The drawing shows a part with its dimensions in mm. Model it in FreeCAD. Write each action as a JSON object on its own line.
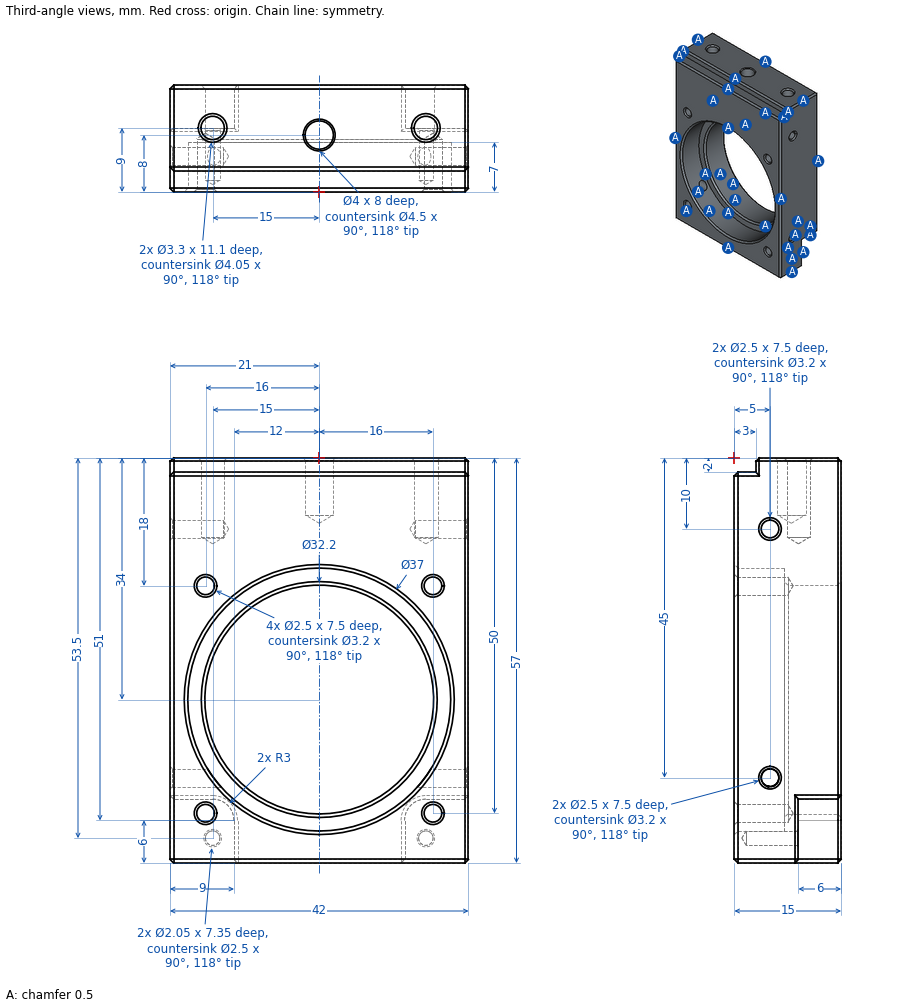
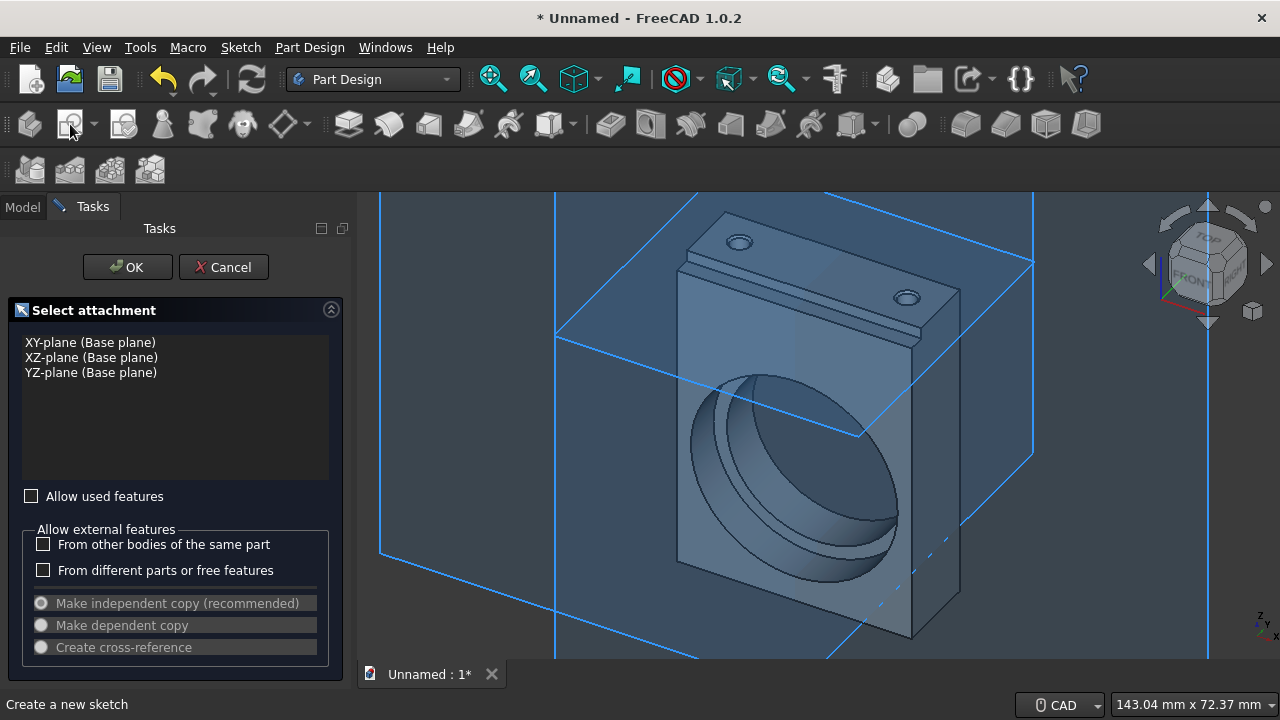
{"action": "left_click", "coordinate": [82, 342]}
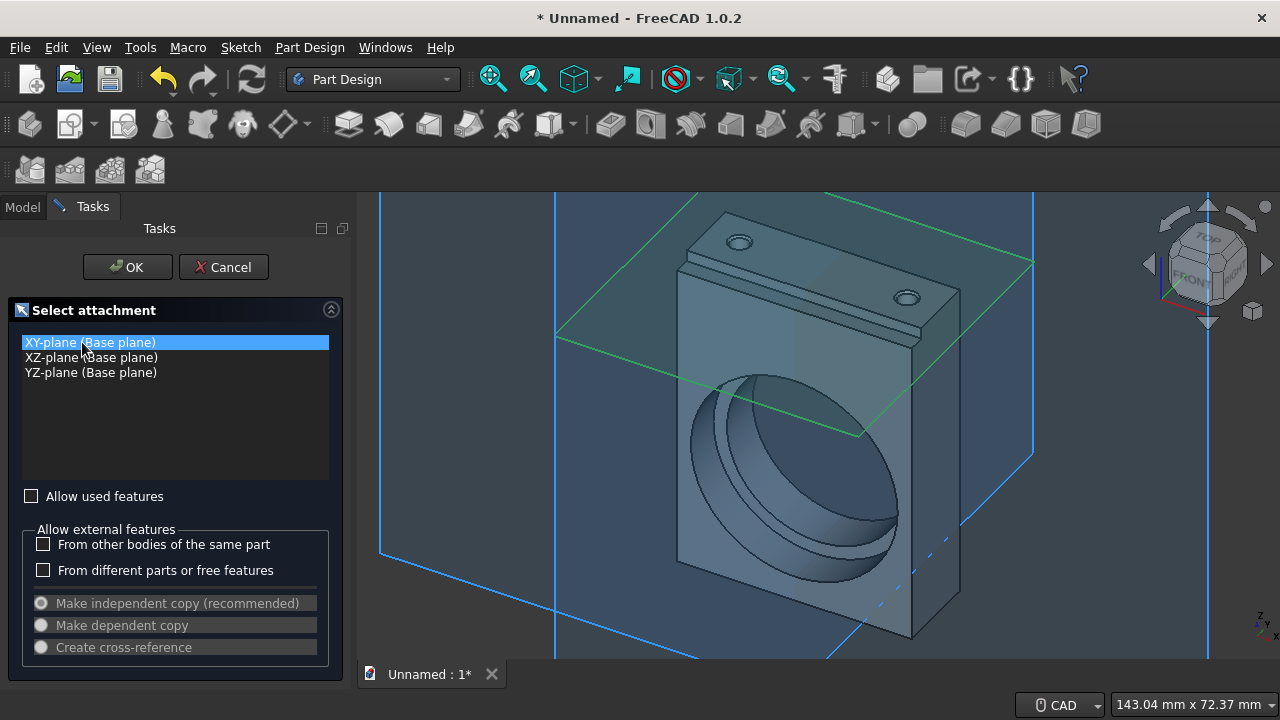
{"action": "left_click", "coordinate": [128, 267]}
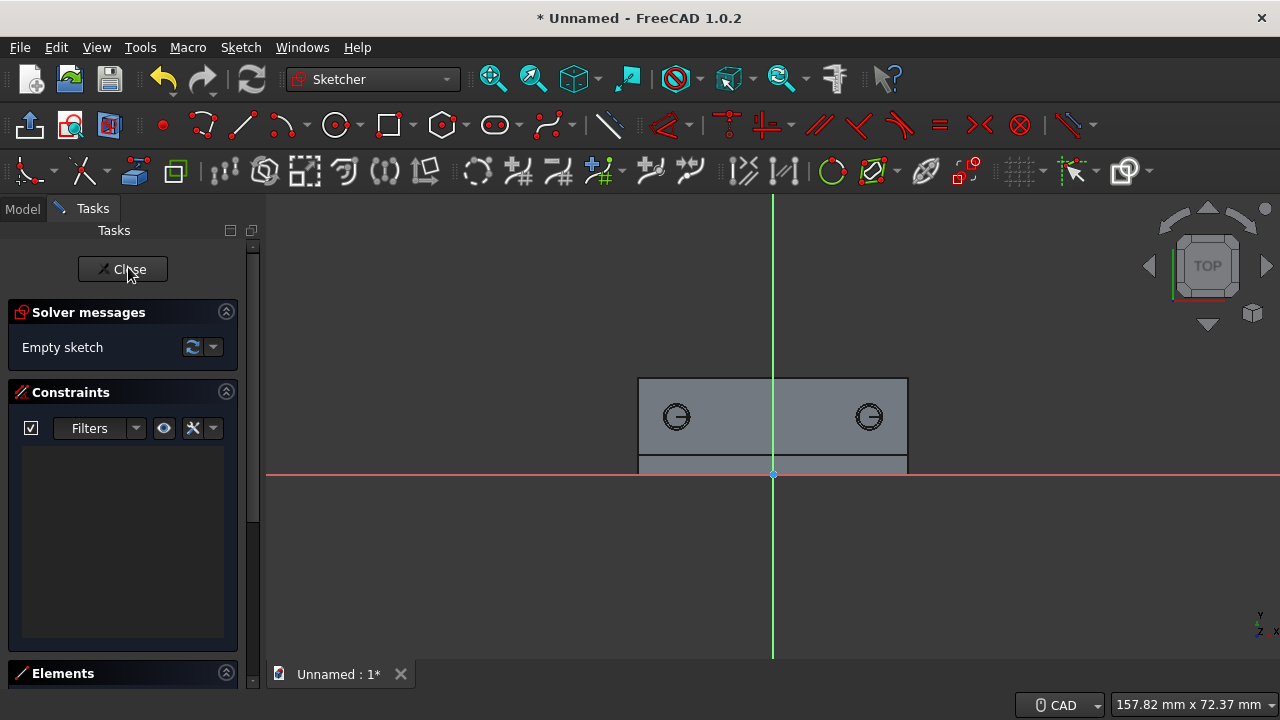
{"action": "scroll", "coordinate": [780, 423], "scroll_direction": "up", "scroll_amount": 12}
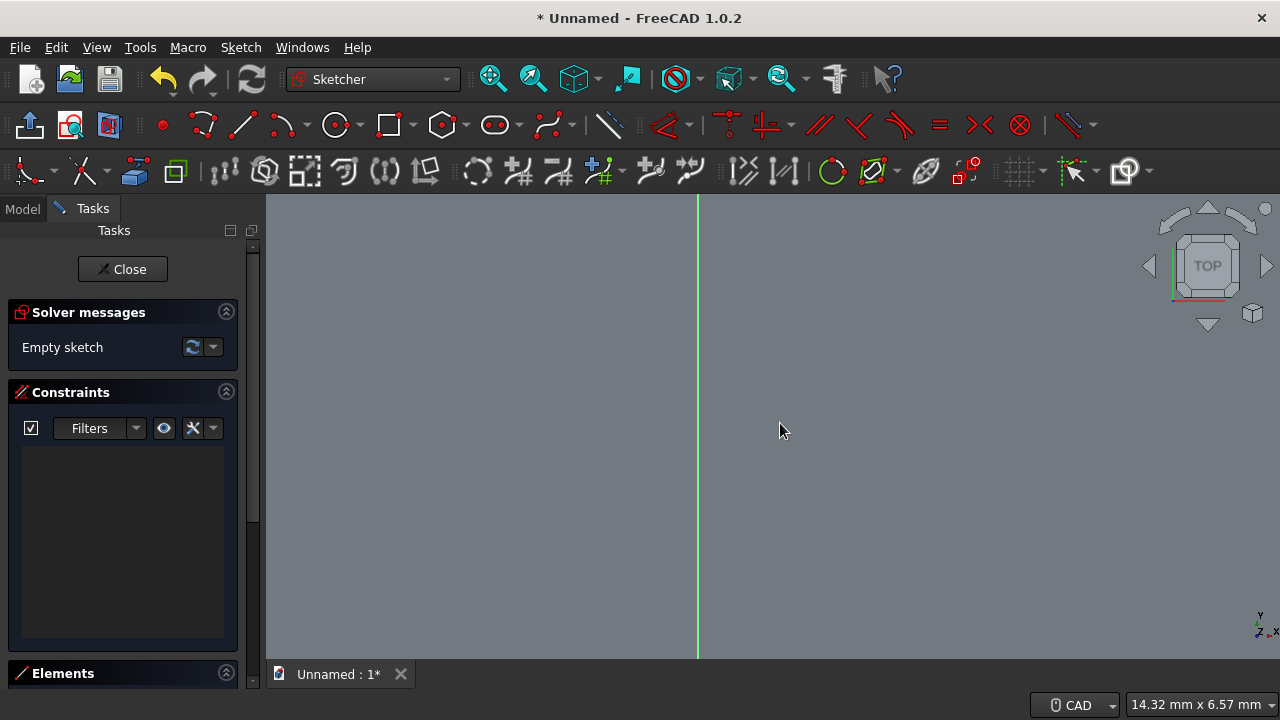
{"action": "key", "text": "g c"}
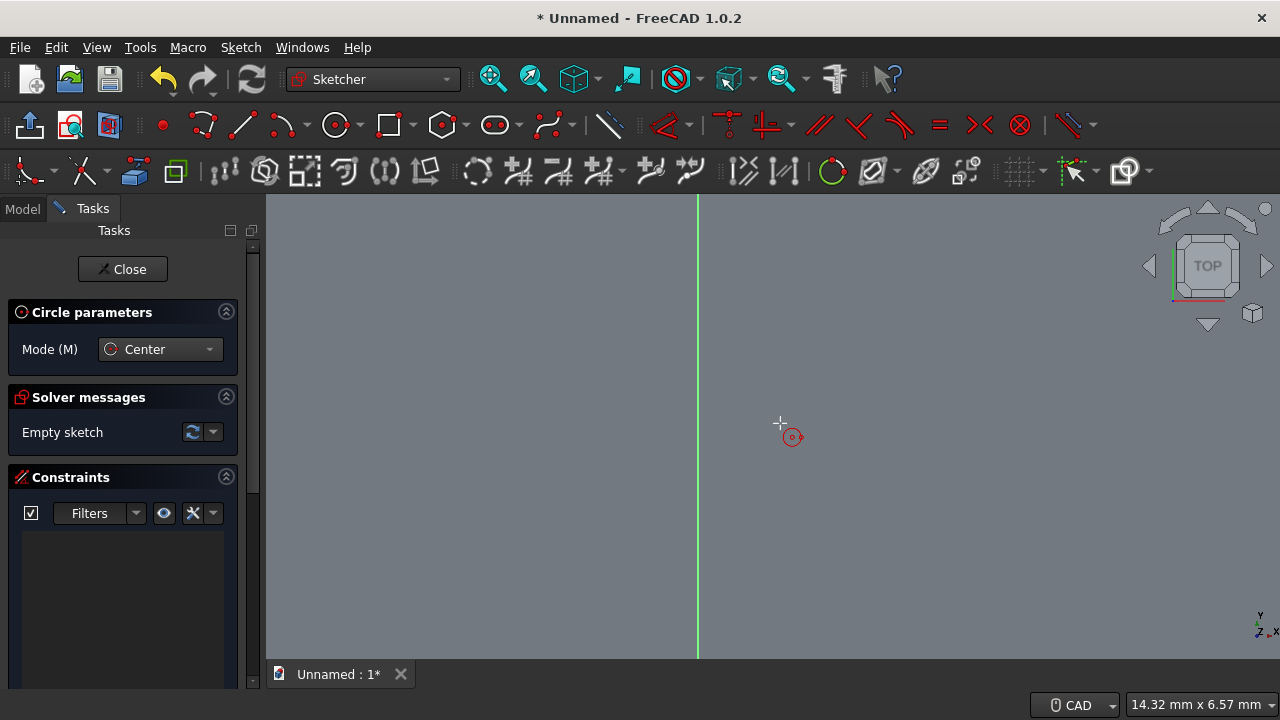
{"action": "left_click", "coordinate": [698, 421]}
{"action": "mouse_move", "coordinate": [798, 321]}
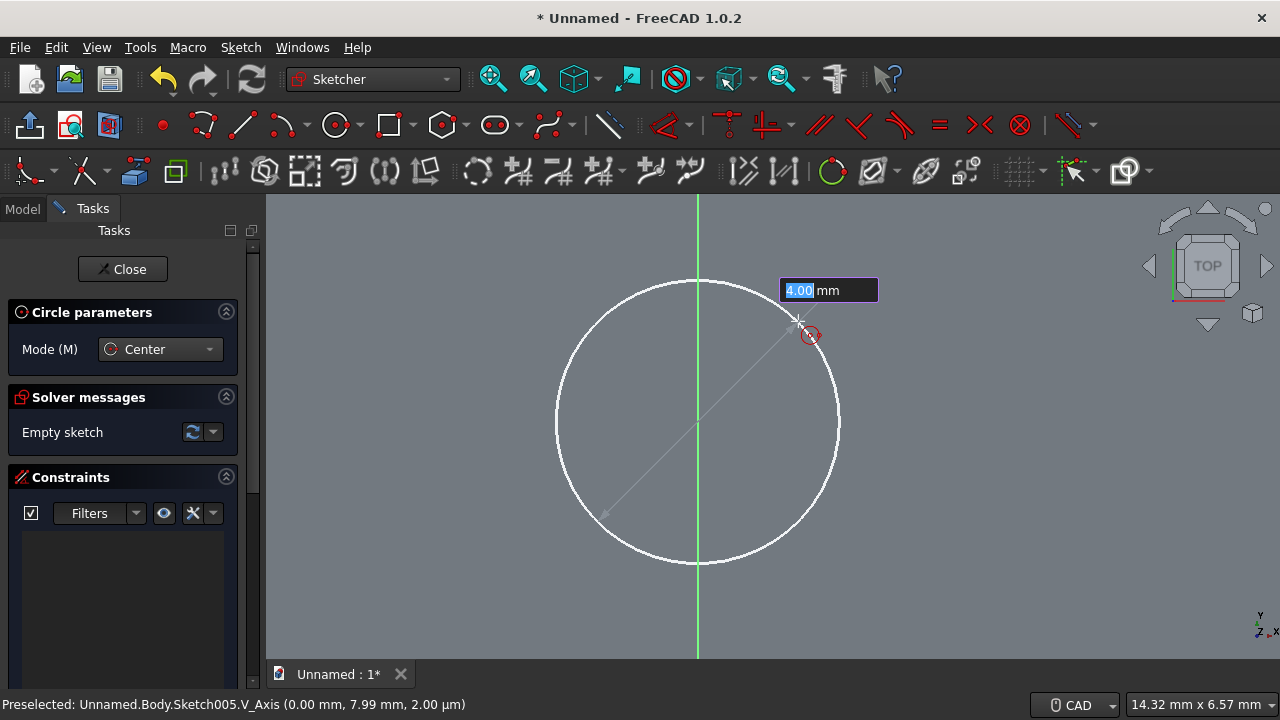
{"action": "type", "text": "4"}
{"action": "key", "text": "Return"}
{"action": "key", "text": "Escape"}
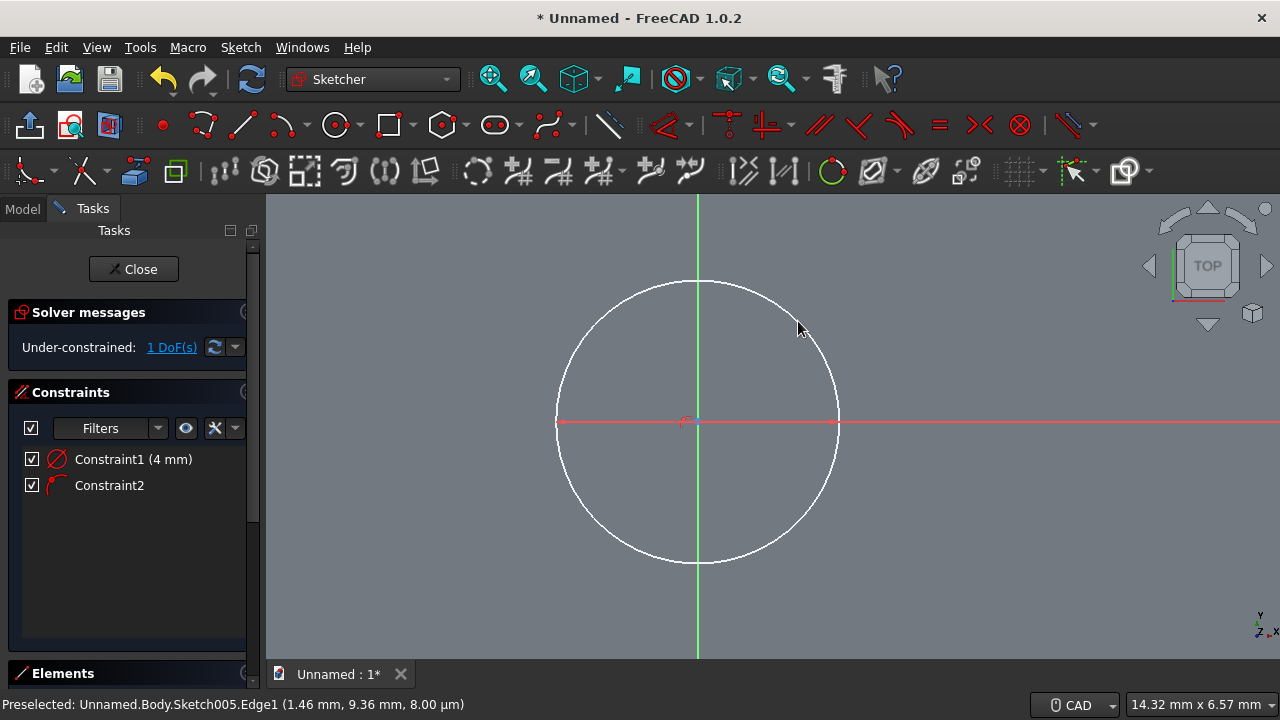
{"action": "key", "text": "d"}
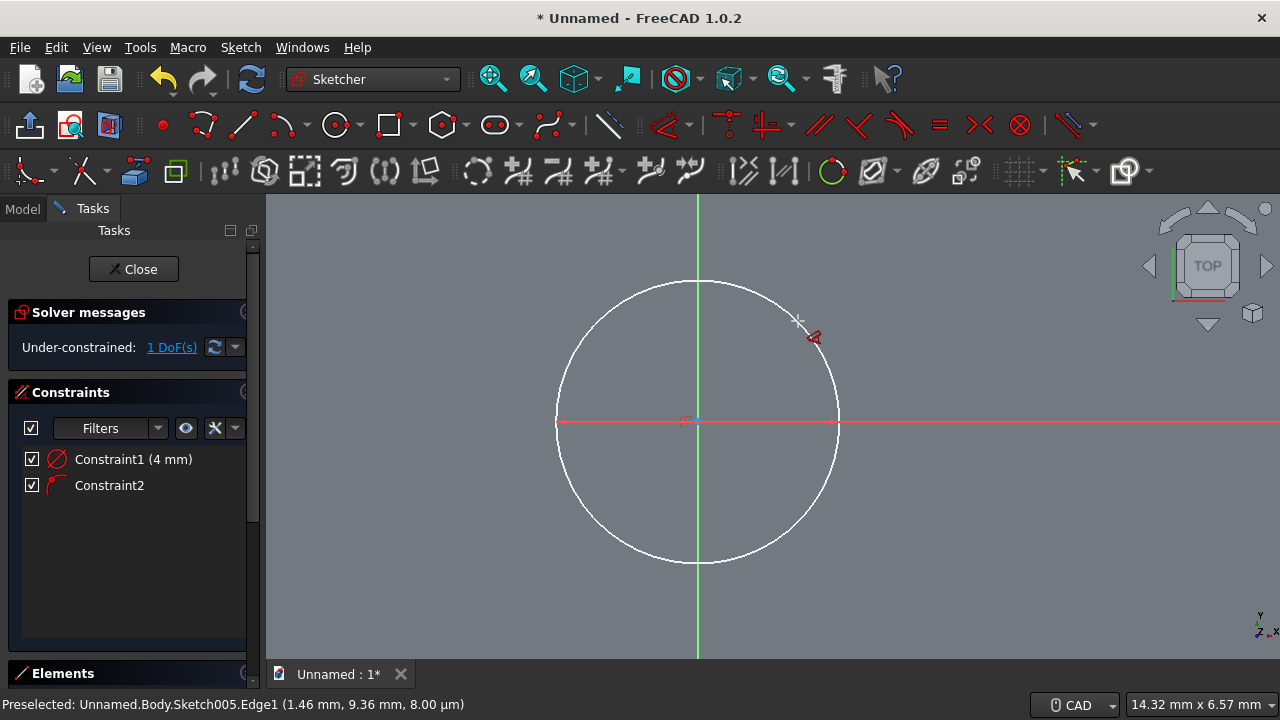
{"action": "left_click", "coordinate": [698, 422]}
{"action": "left_click", "coordinate": [732, 526]}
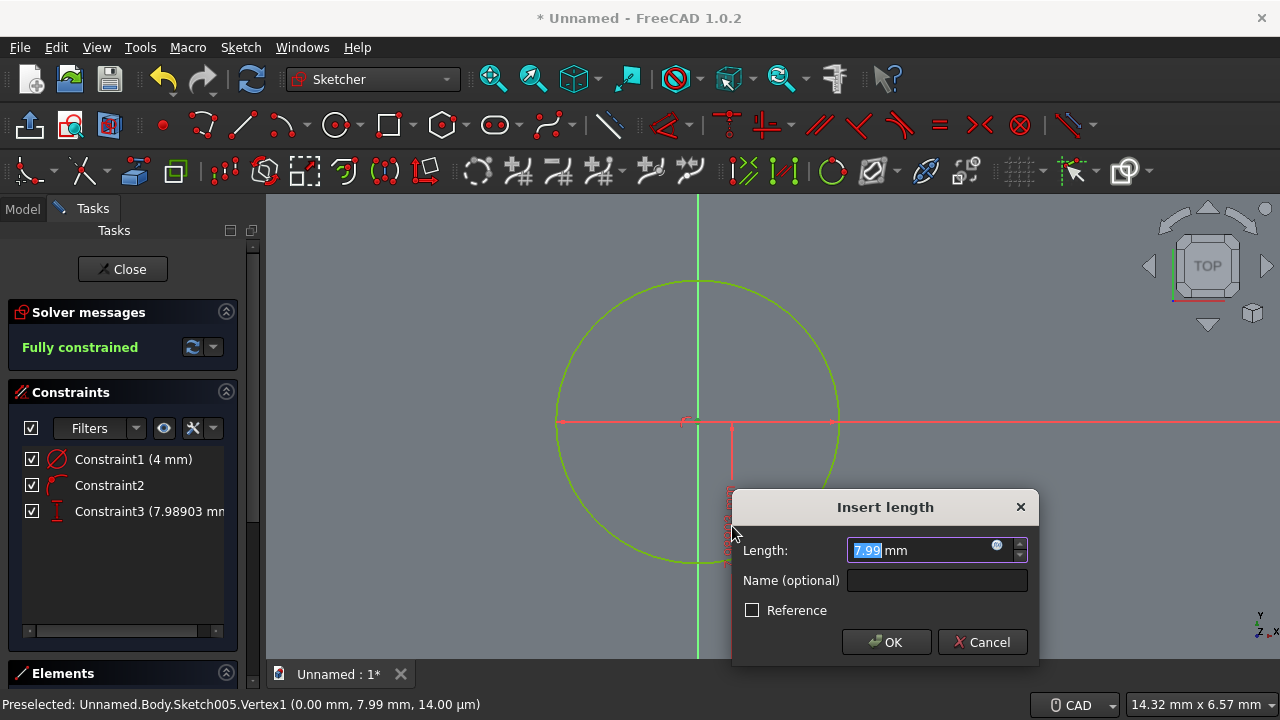
{"action": "type", "text": "8"}
{"action": "key", "text": "Return"}
{"action": "key", "text": "Escape"}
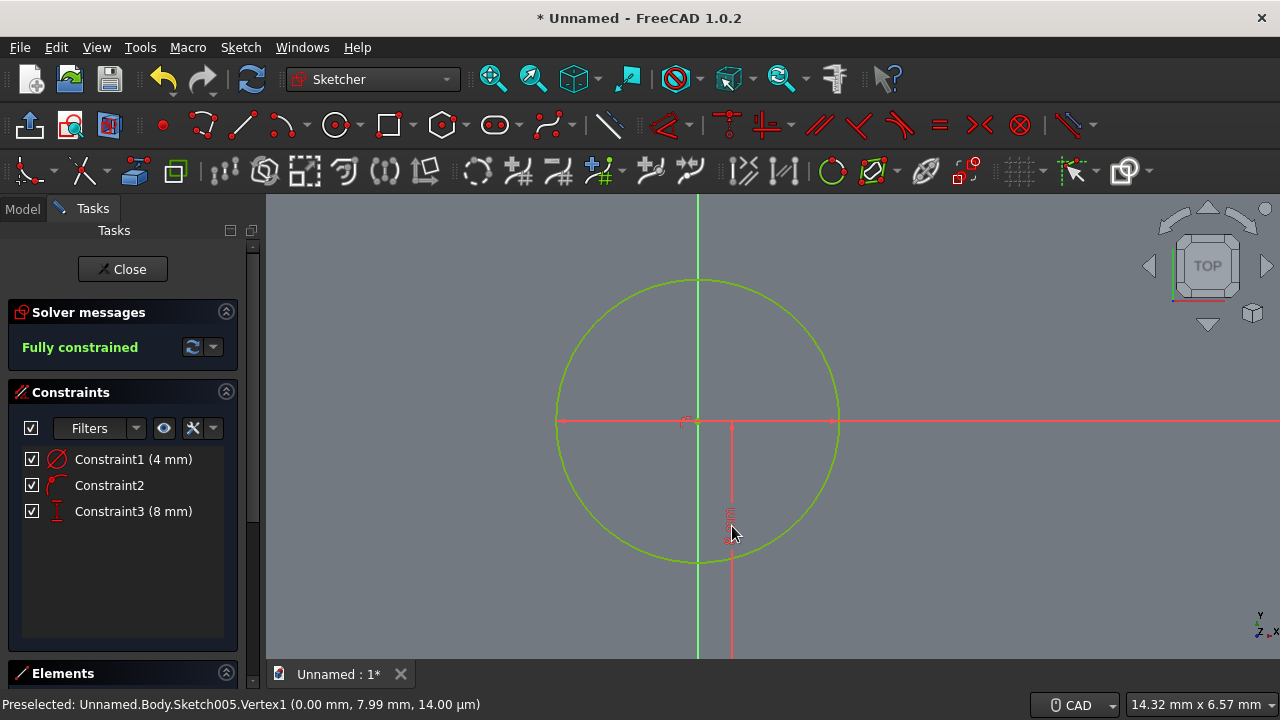
{"action": "left_click", "coordinate": [123, 269]}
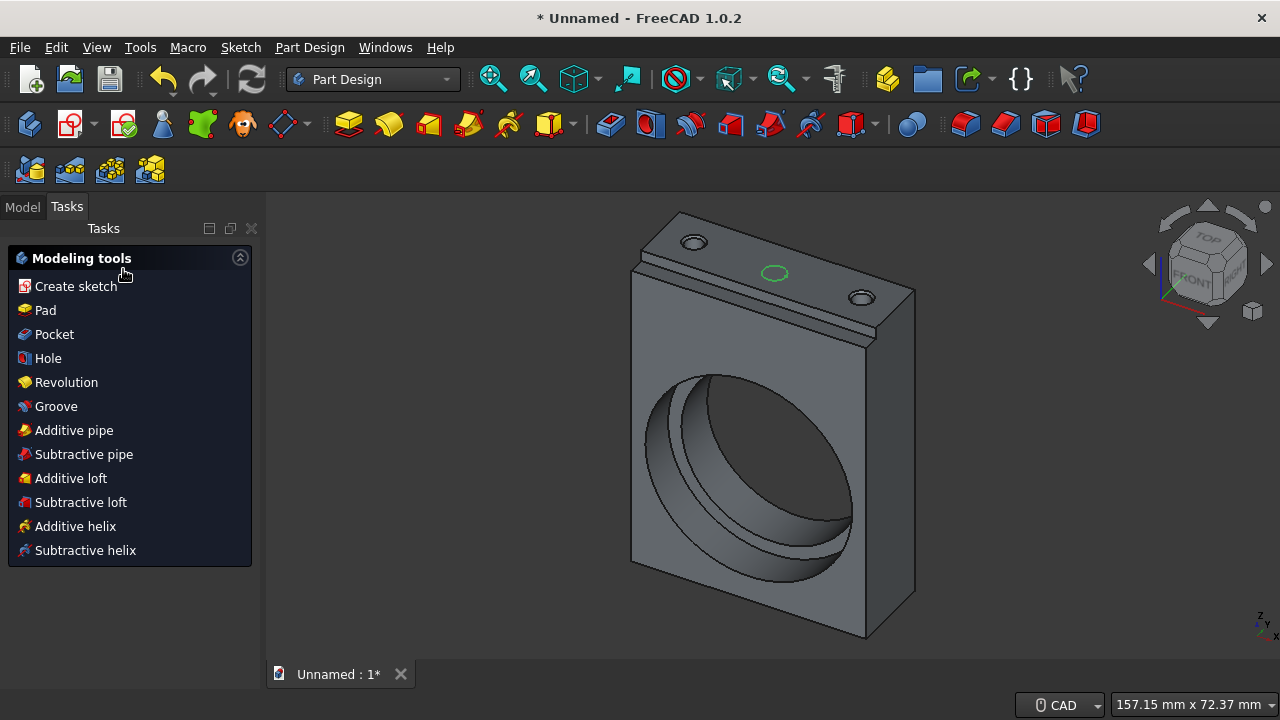
{"action": "left_click", "coordinate": [652, 124]}